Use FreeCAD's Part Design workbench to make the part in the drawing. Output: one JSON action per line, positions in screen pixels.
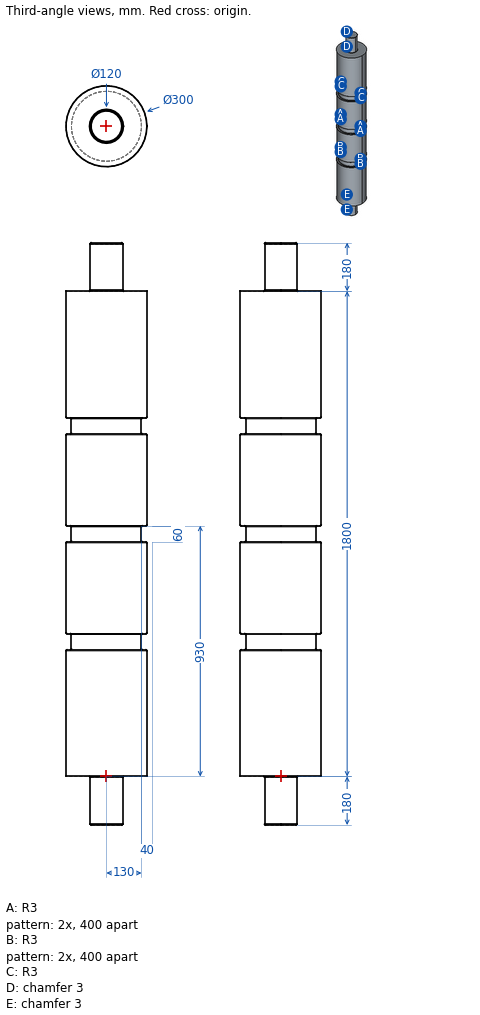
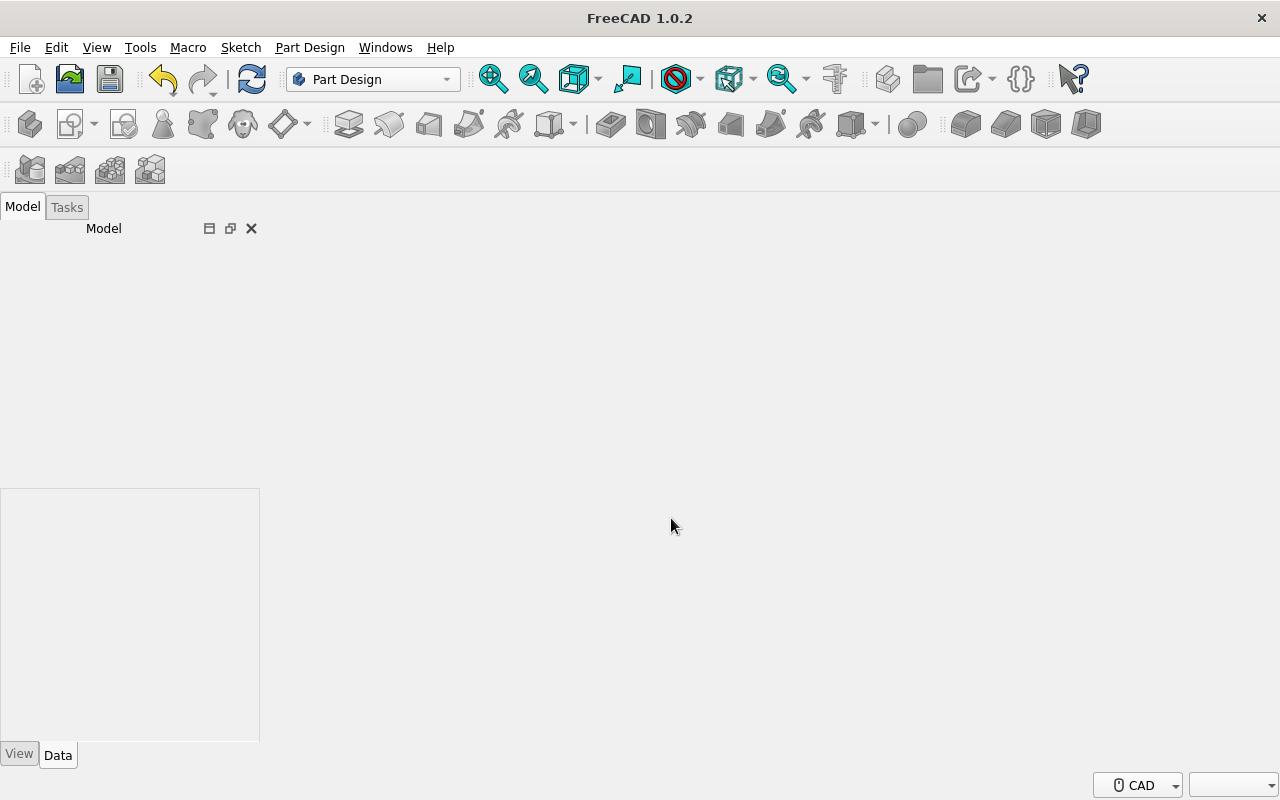
{"action": "left_click", "coordinate": [30, 80]}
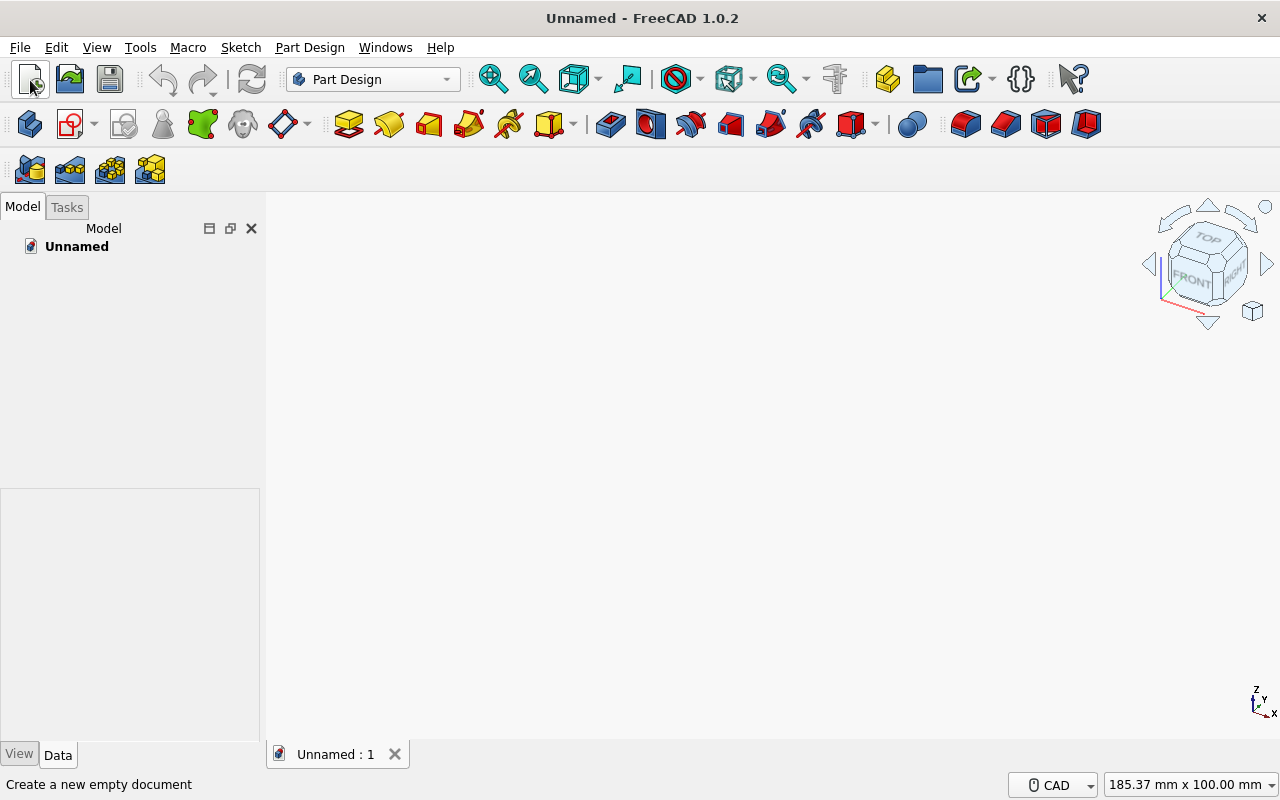
{"action": "left_click", "coordinate": [70, 124]}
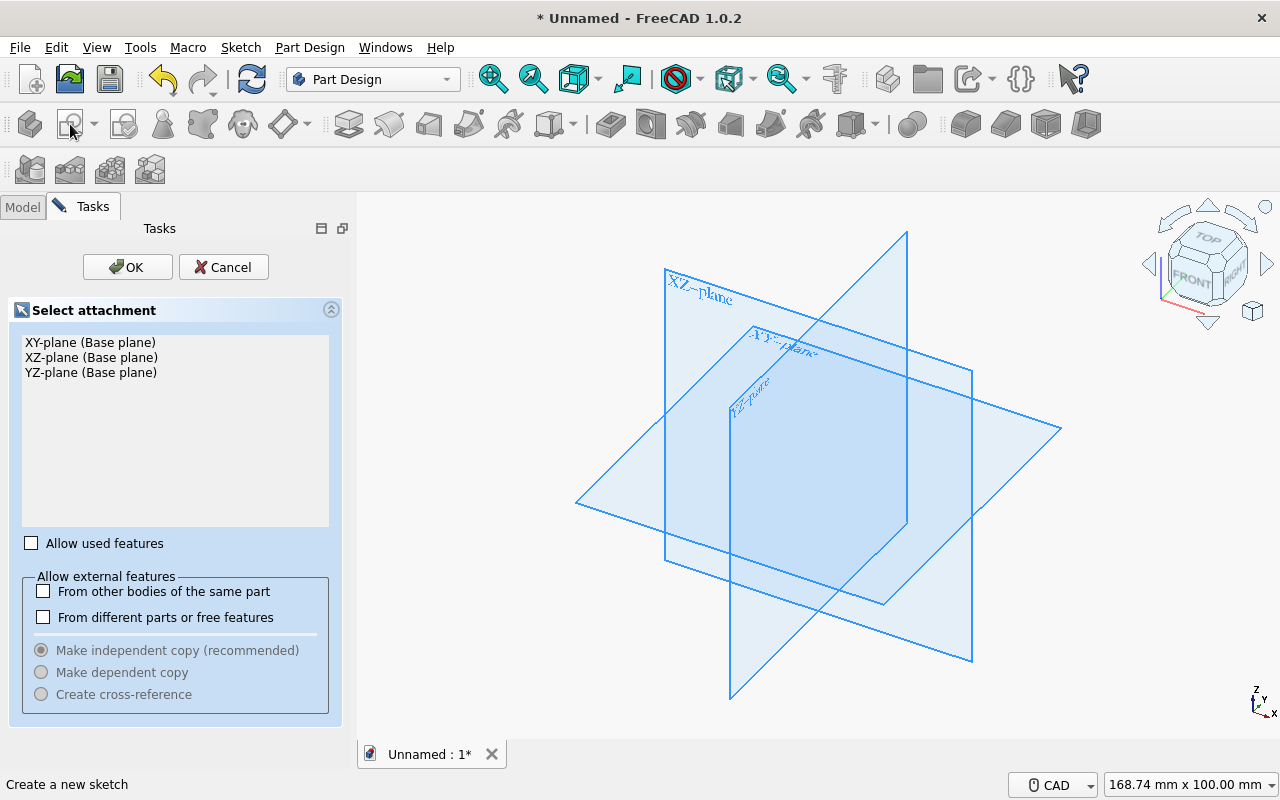
{"action": "left_click", "coordinate": [82, 342]}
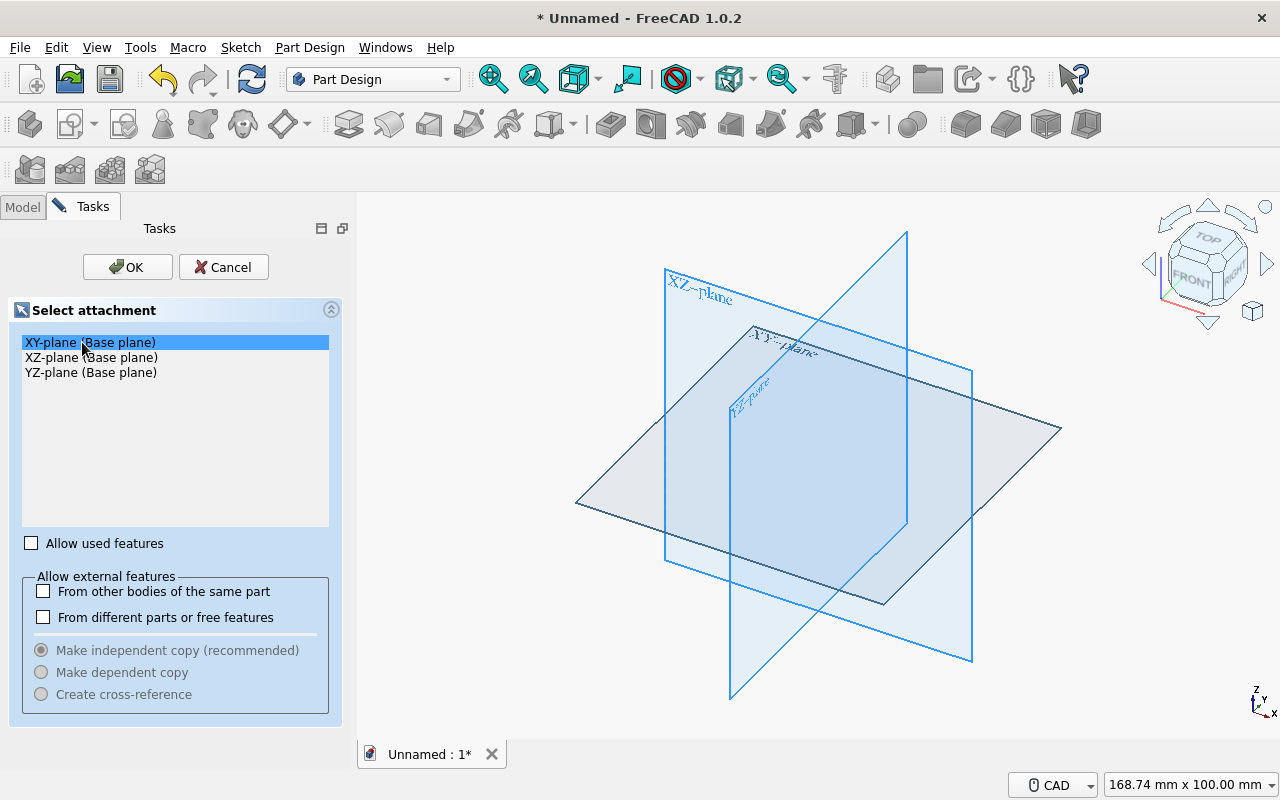
{"action": "left_click", "coordinate": [128, 267]}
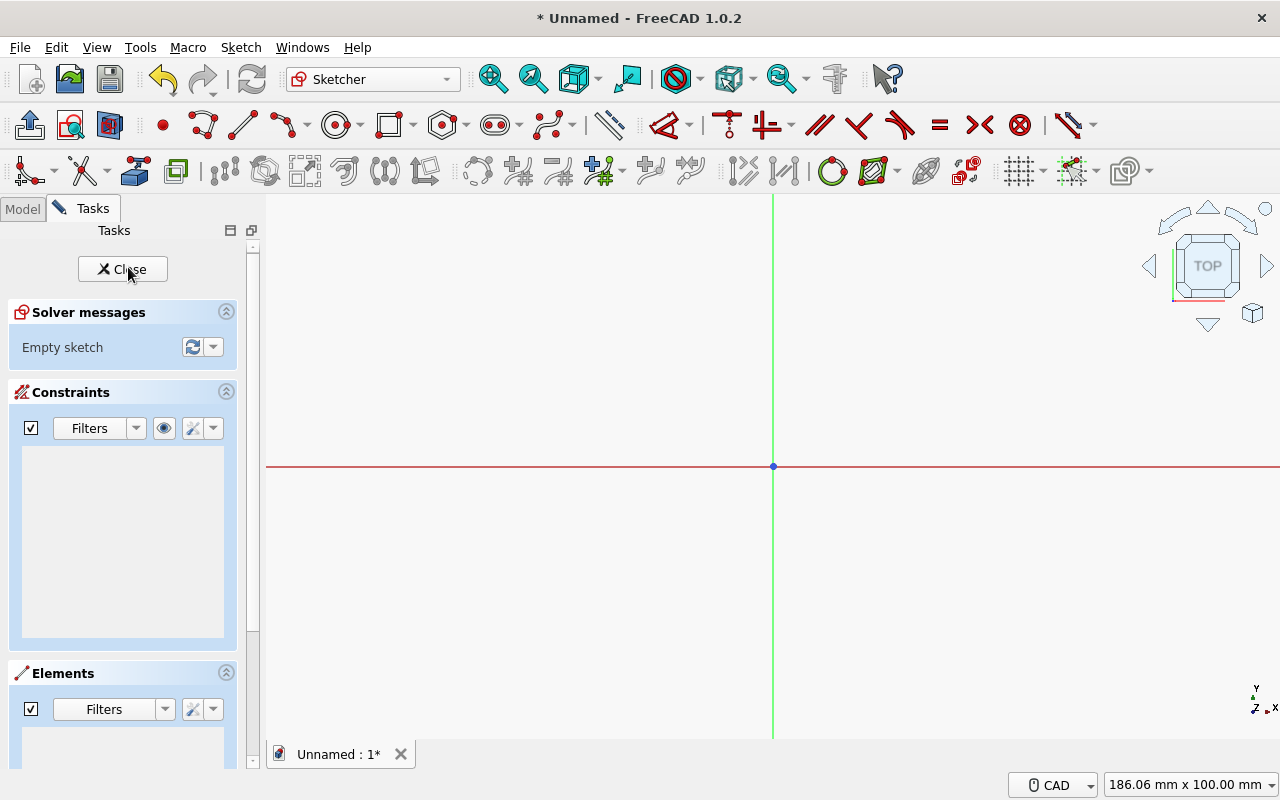
{"action": "scroll", "coordinate": [687, 466], "scroll_direction": "down", "scroll_amount": 8}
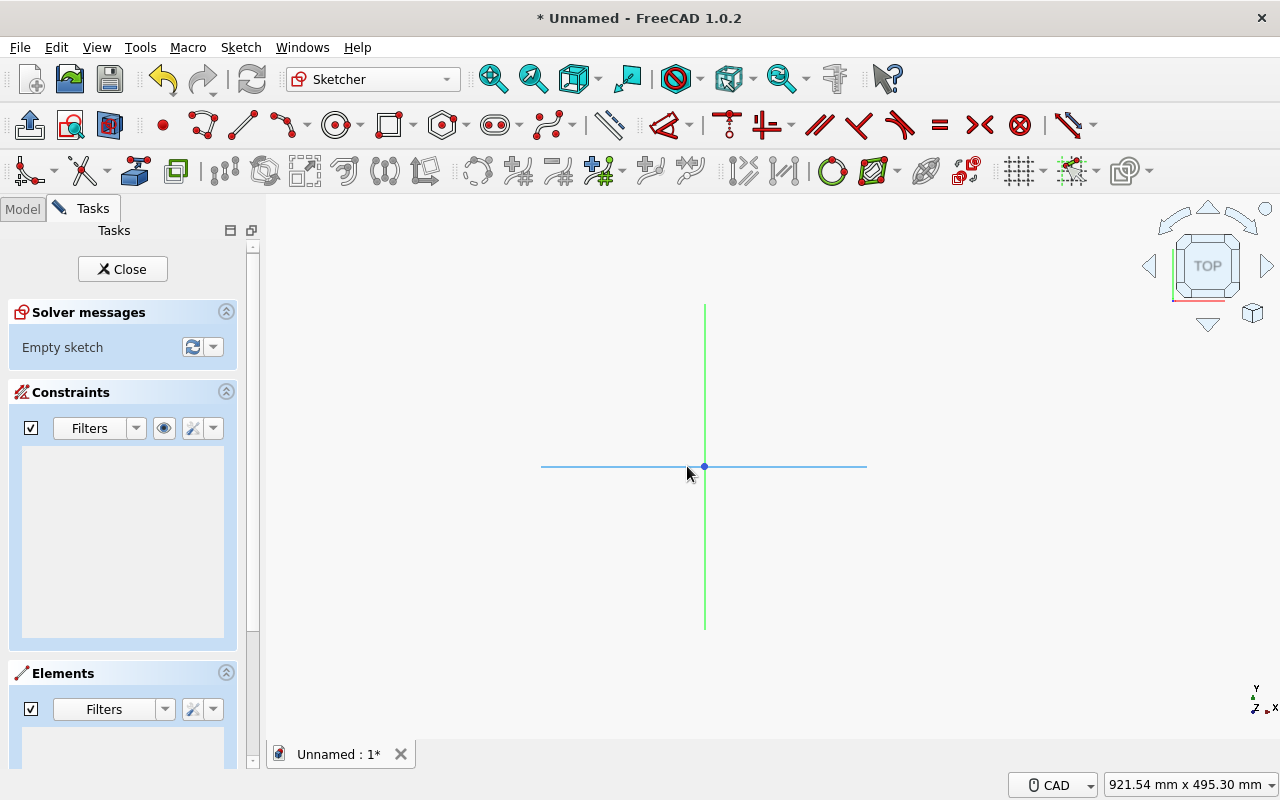
{"action": "left_click", "coordinate": [336, 126]}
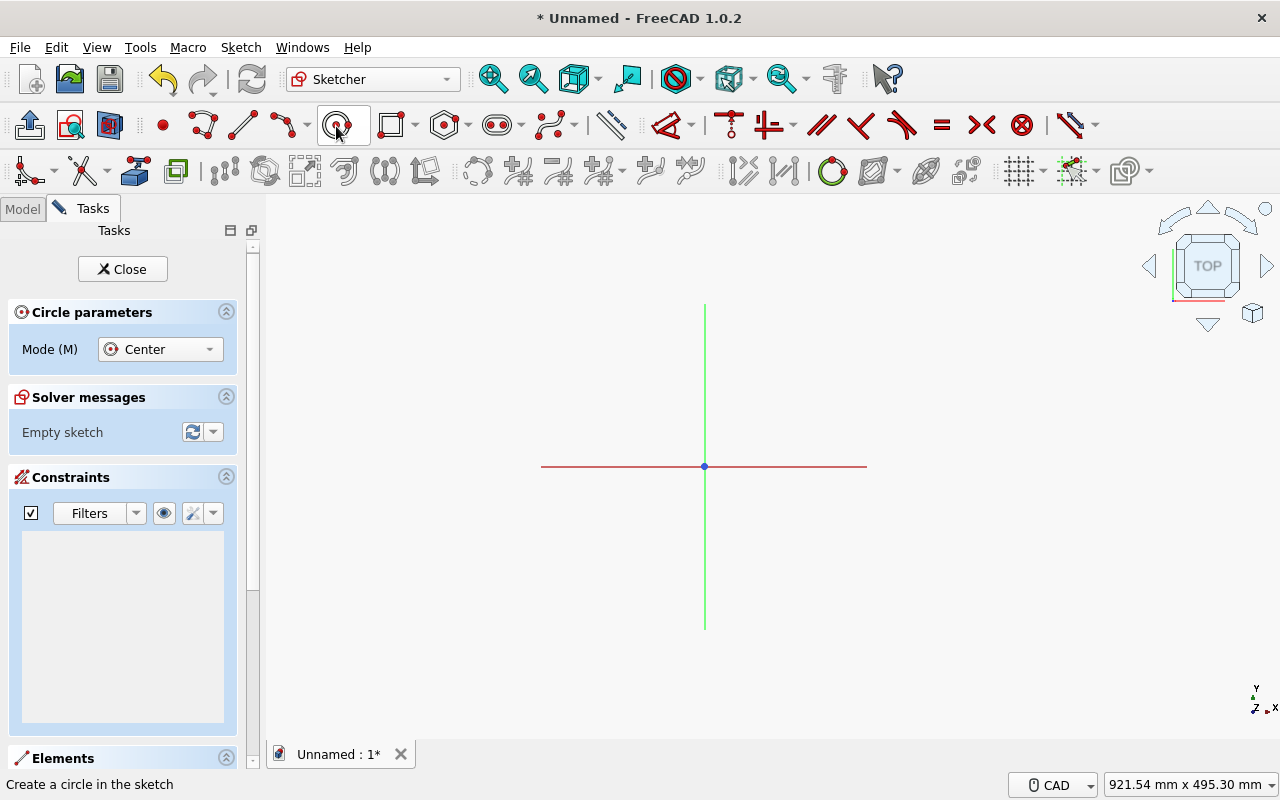
{"action": "left_click", "coordinate": [705, 466]}
{"action": "mouse_move", "coordinate": [821, 350]}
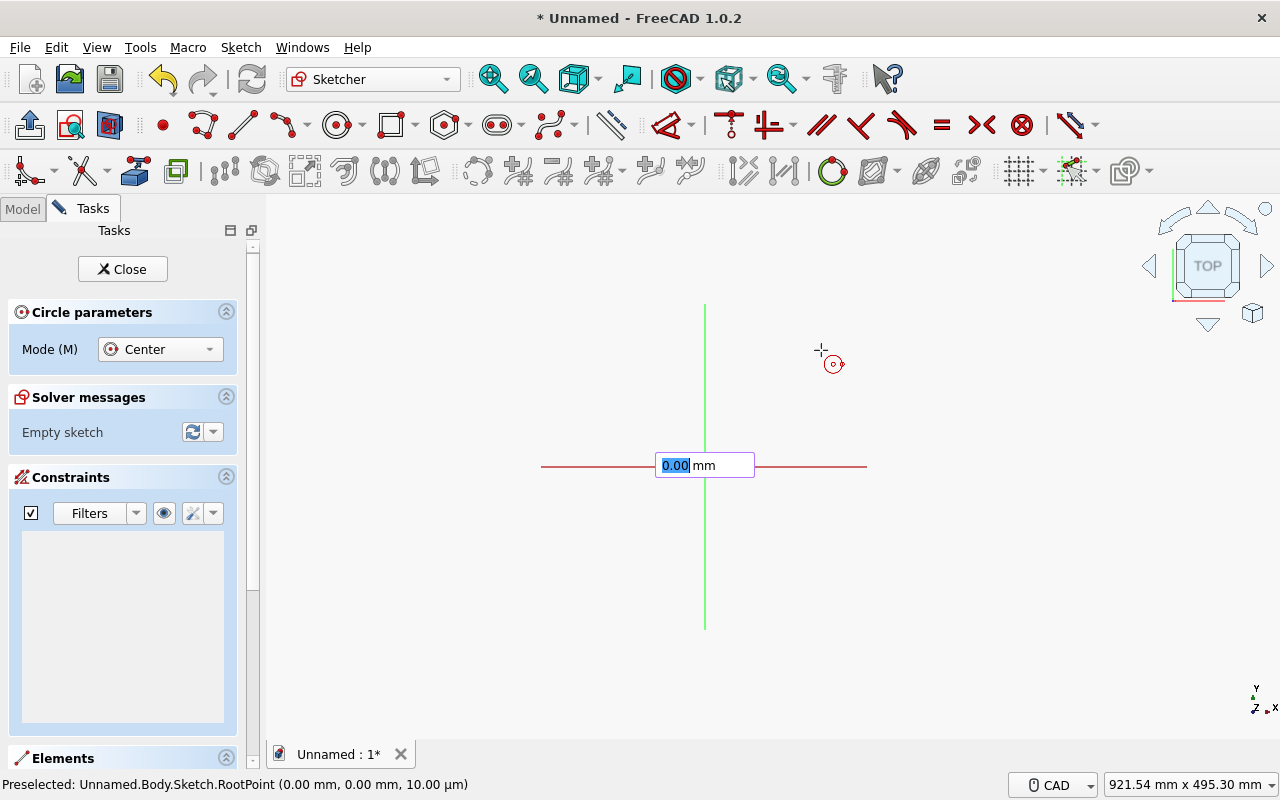
{"action": "type", "text": "300"}
{"action": "key", "text": "Return"}
{"action": "key", "text": "Escape"}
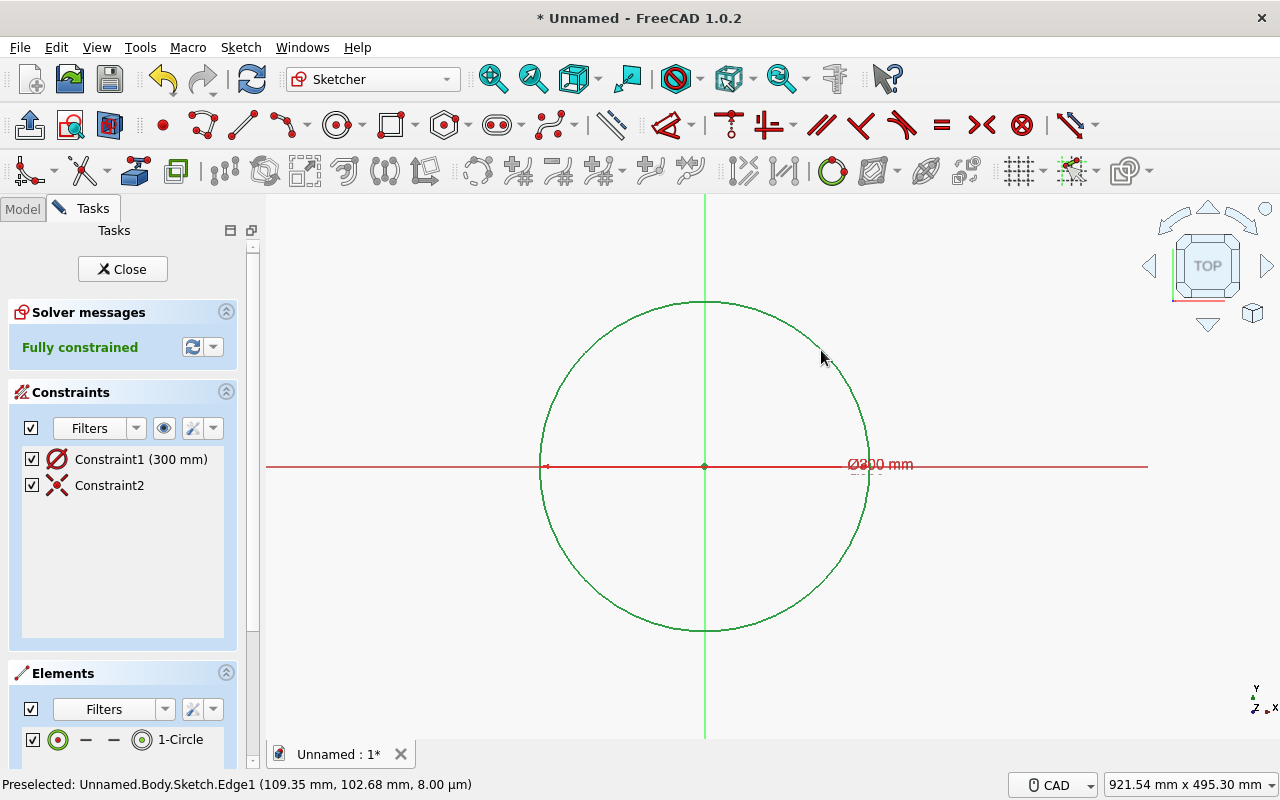
{"action": "left_click", "coordinate": [123, 269]}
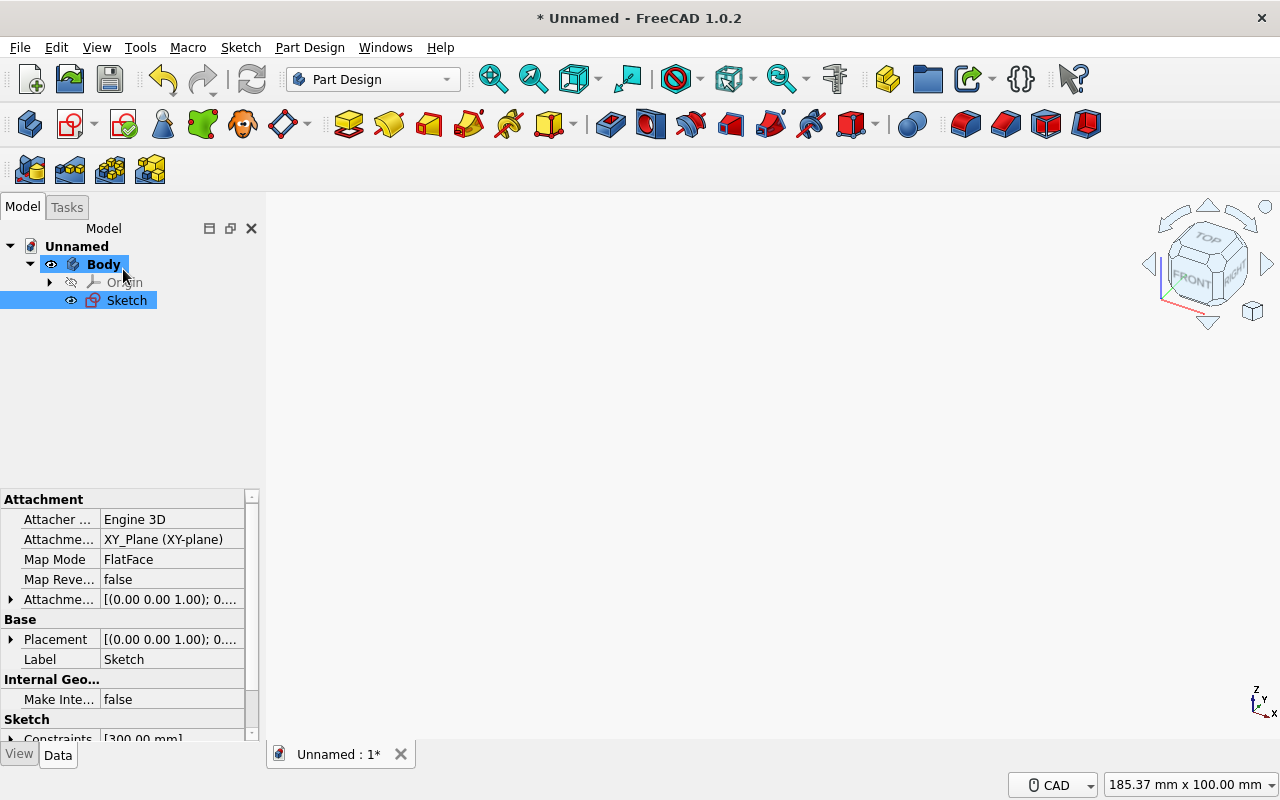
{"action": "left_click", "coordinate": [350, 124]}